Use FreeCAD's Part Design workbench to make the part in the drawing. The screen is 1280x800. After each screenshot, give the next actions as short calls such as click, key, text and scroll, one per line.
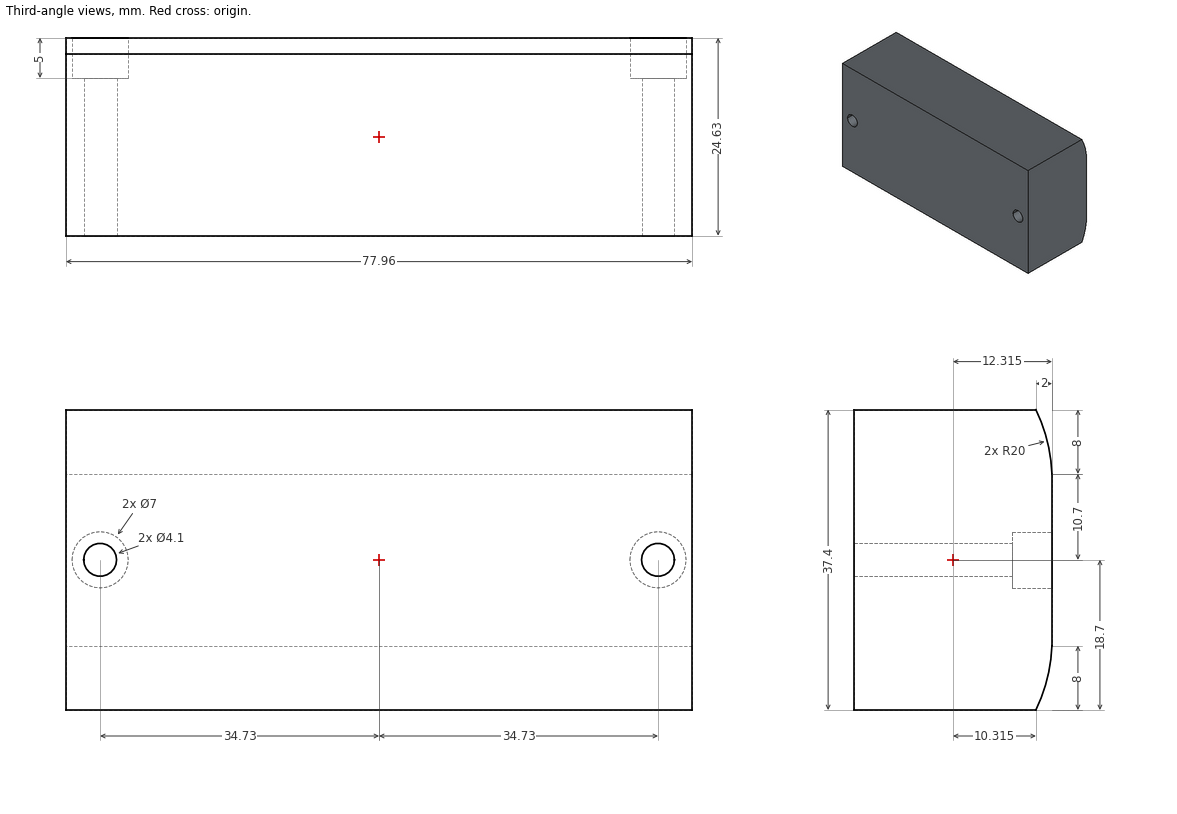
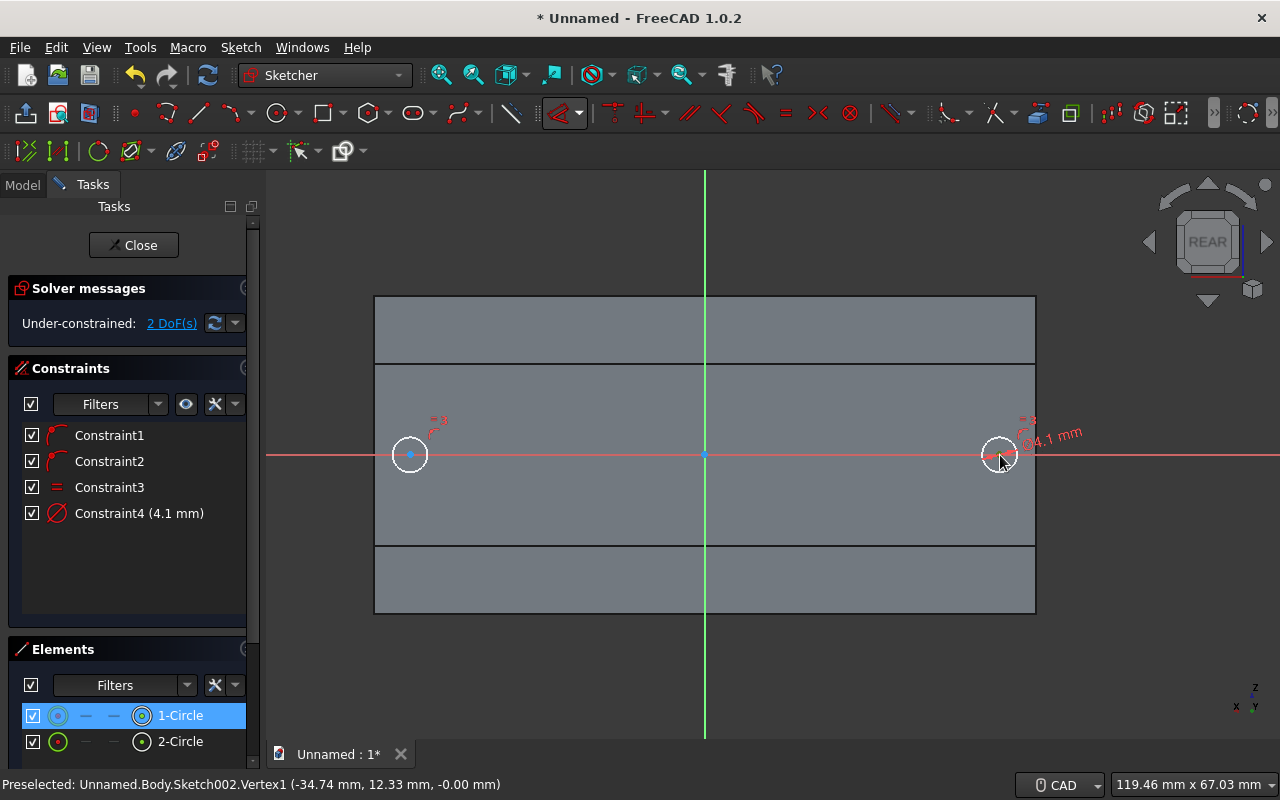
key(l)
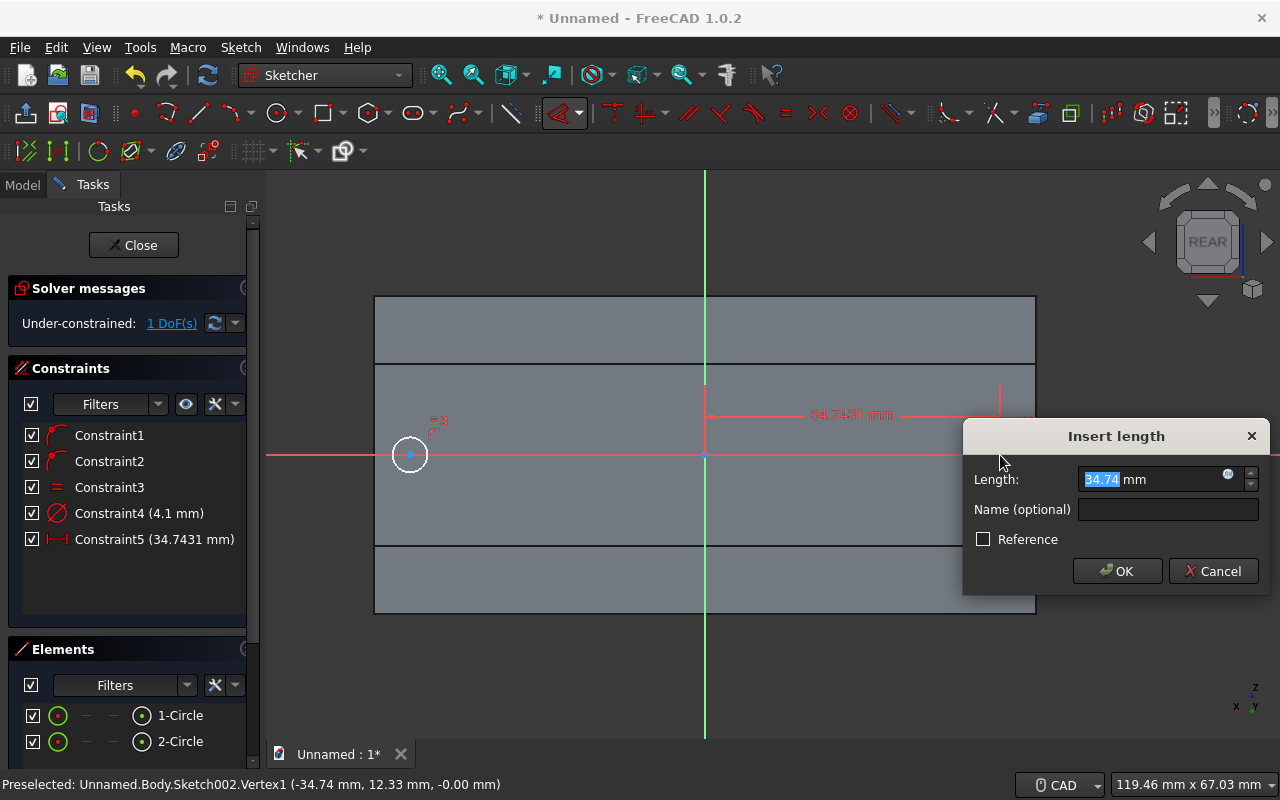
text(34.73)
key(Return)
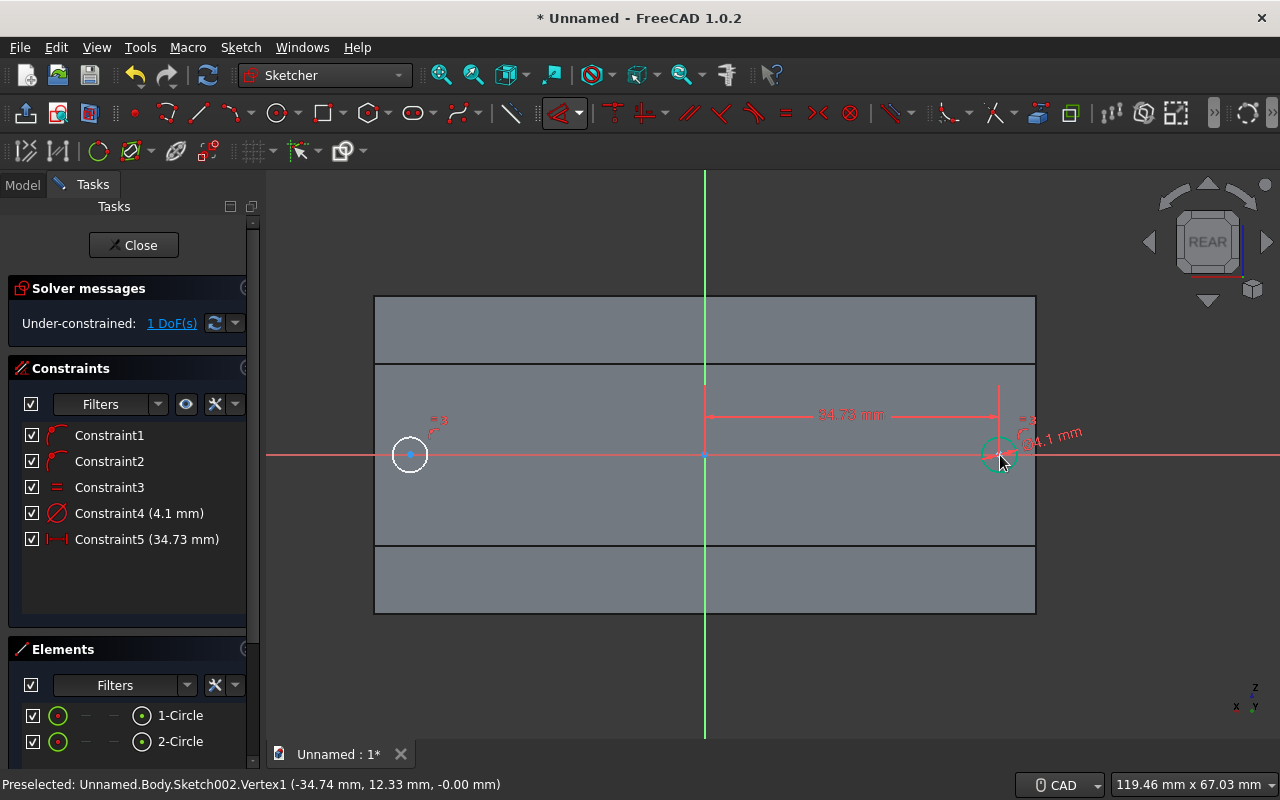
click(410, 455)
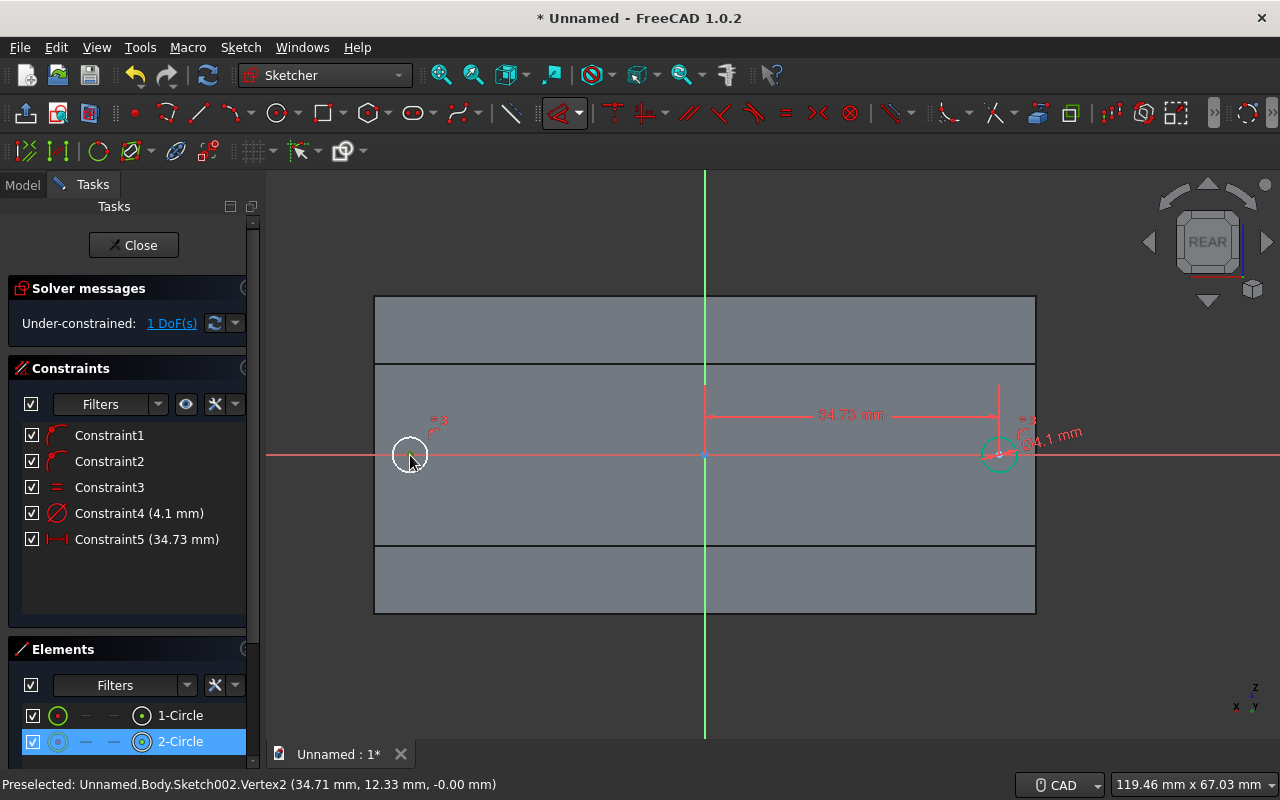
key(l)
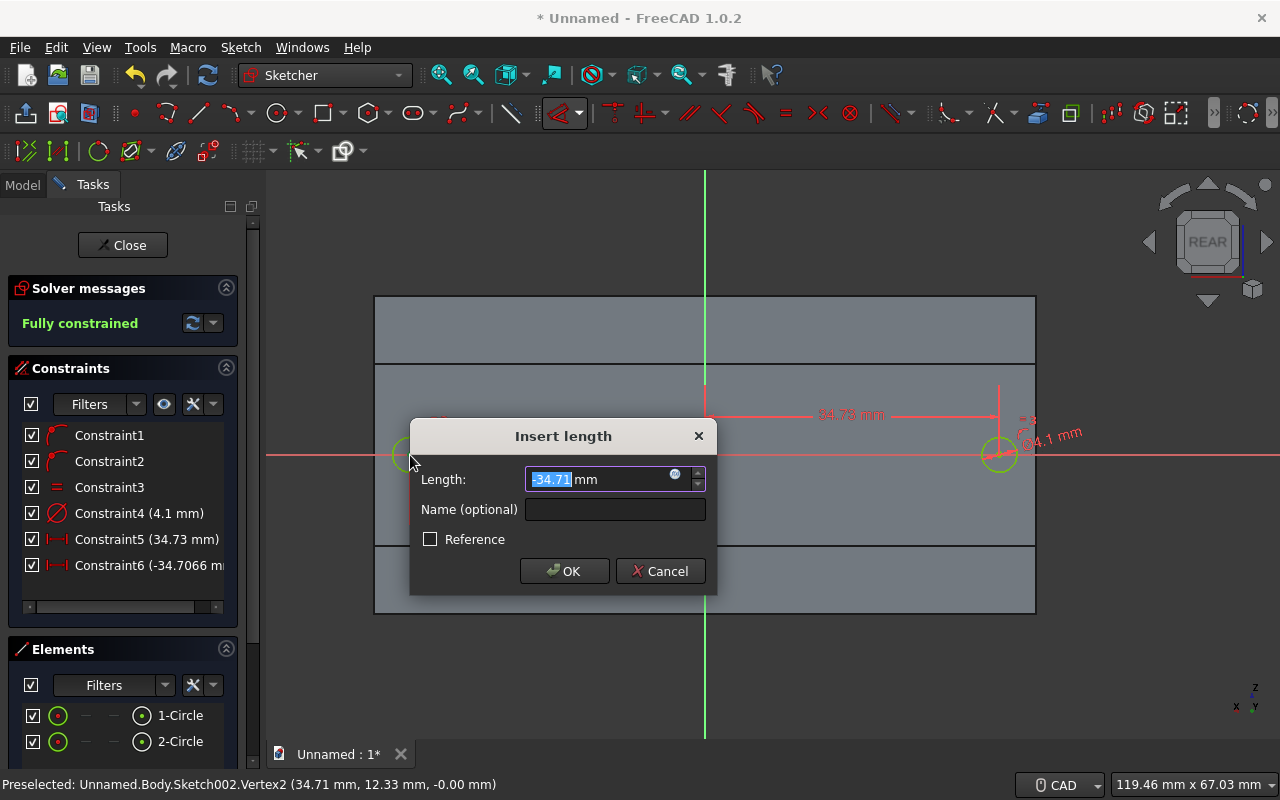
text(-34.73)
key(Return)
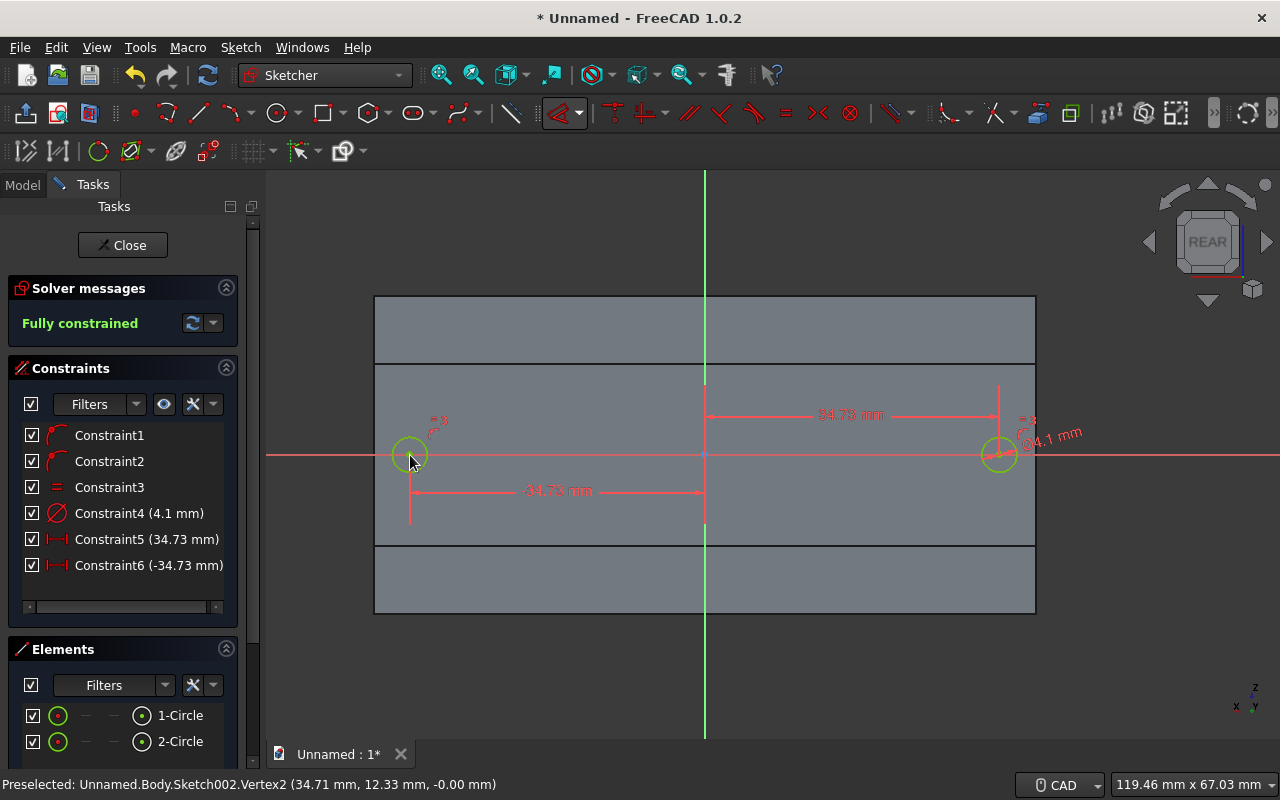
click(123, 245)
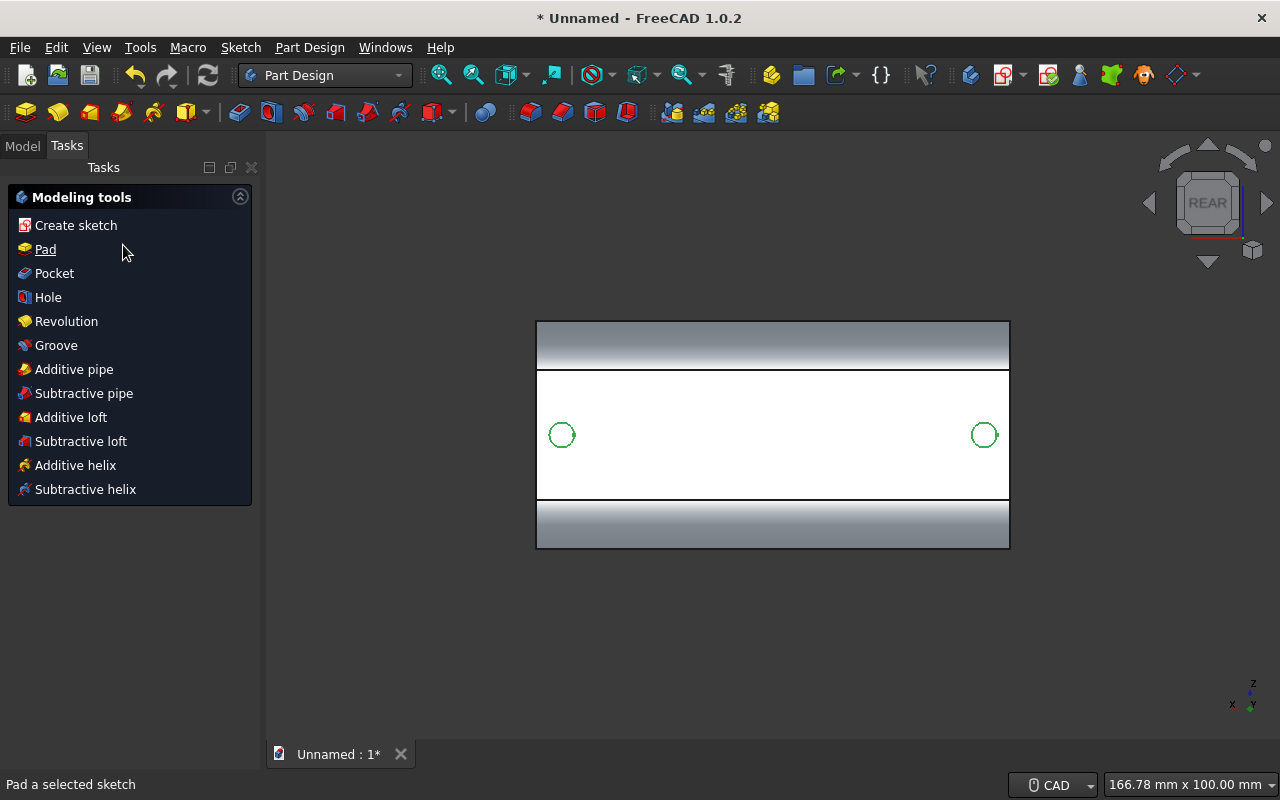
click(240, 112)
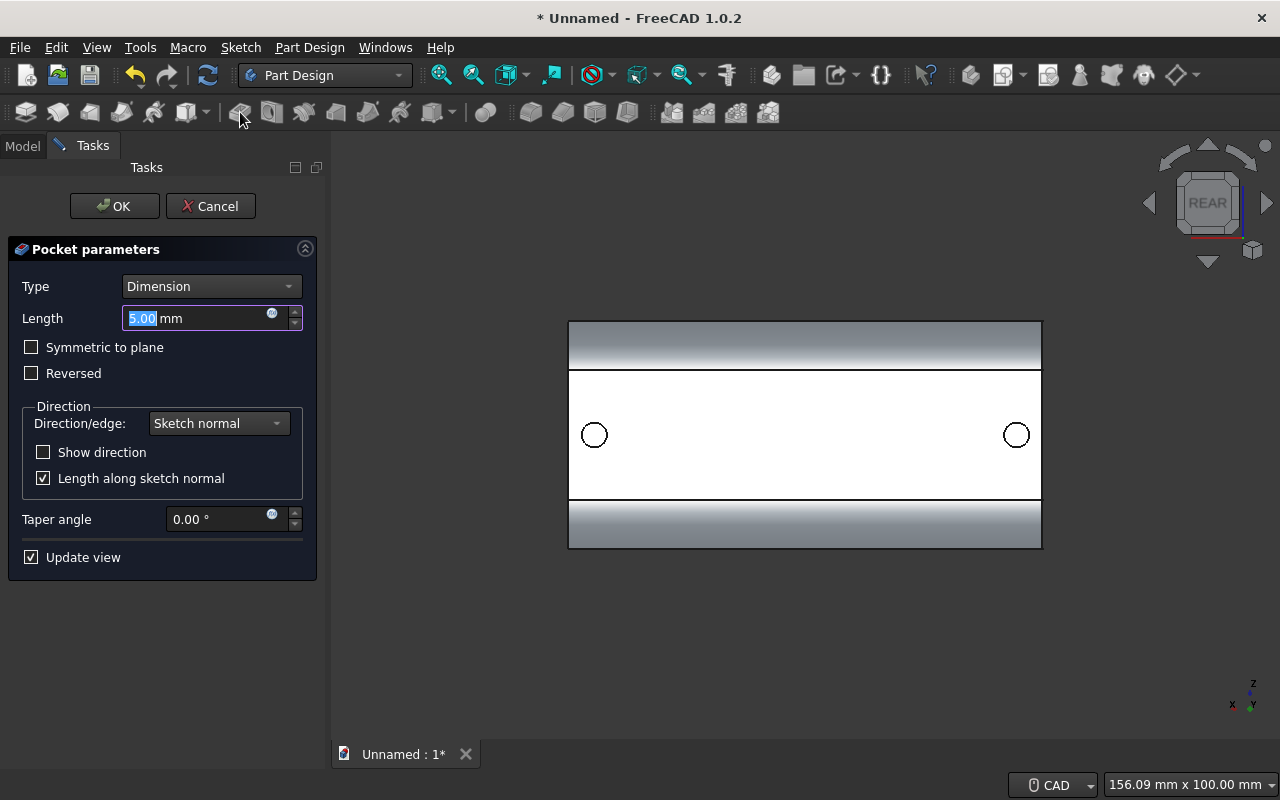
click(212, 286)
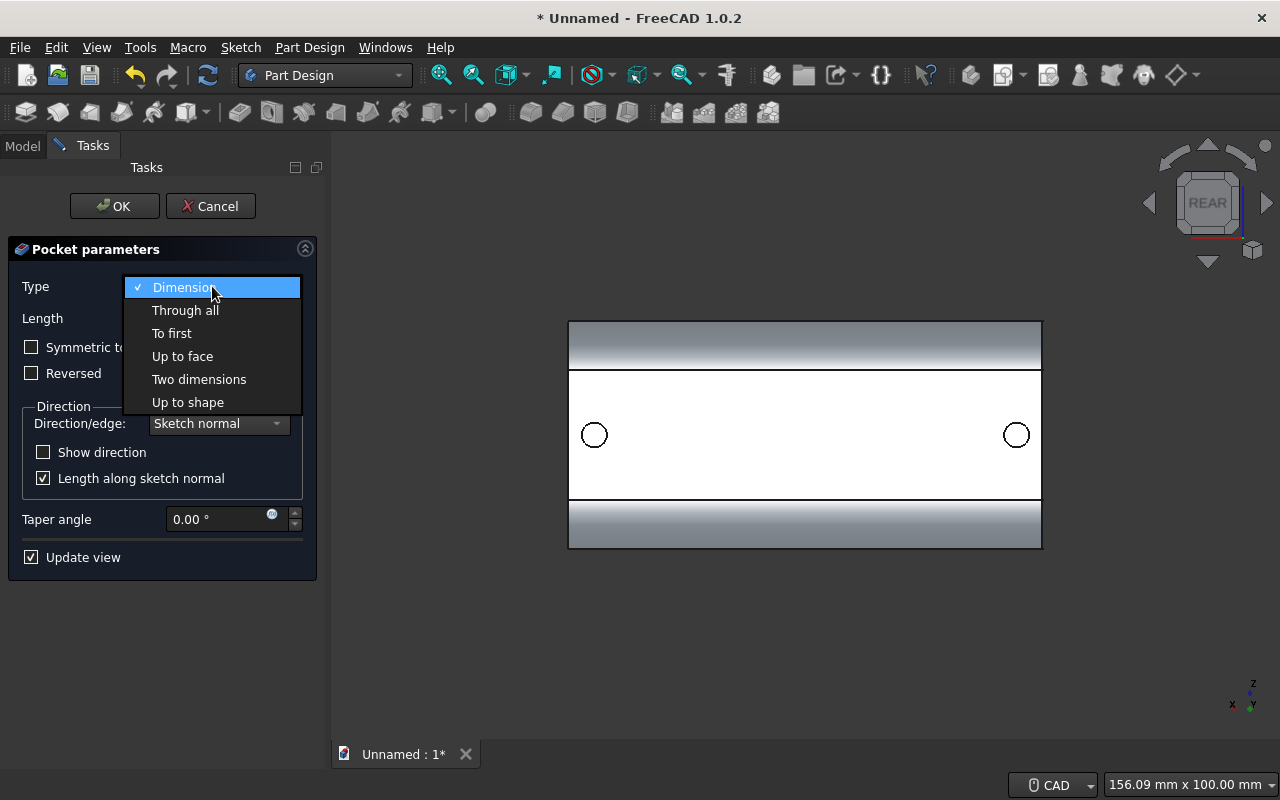
click(212, 310)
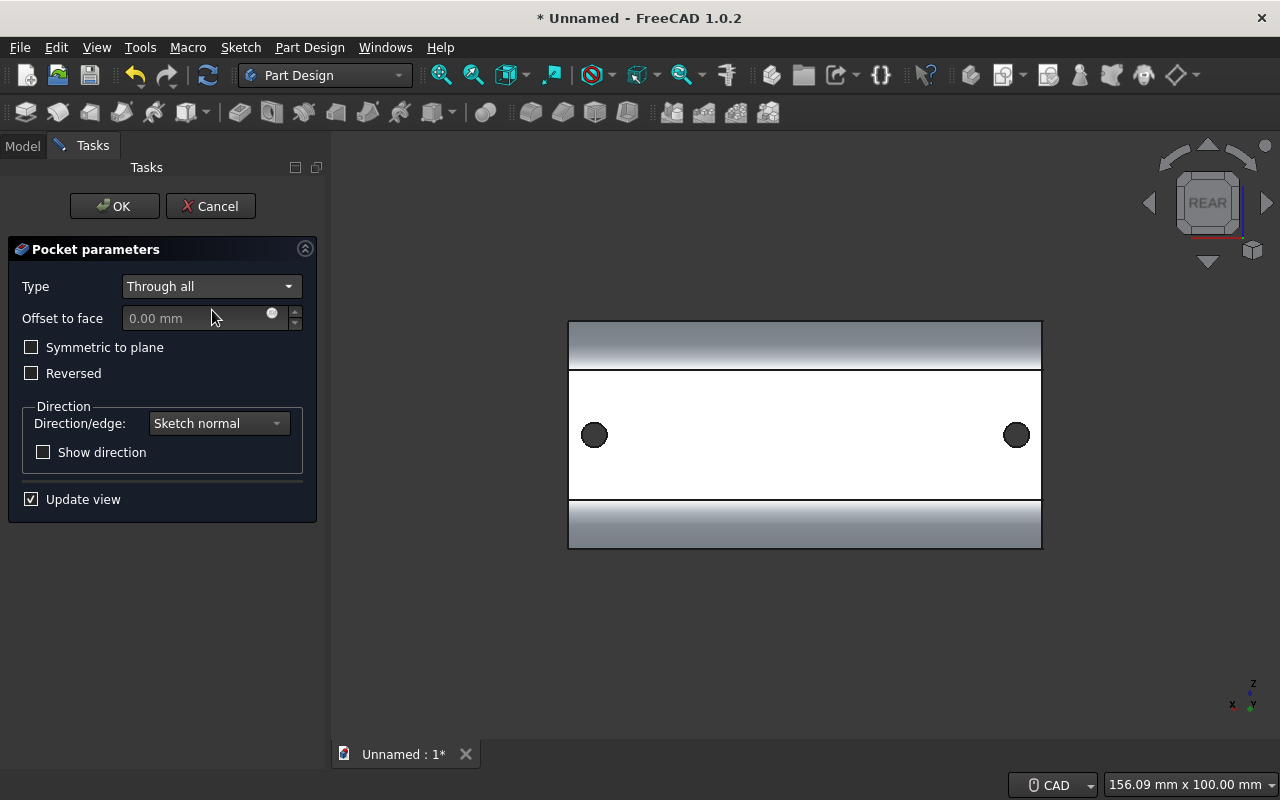
click(115, 206)